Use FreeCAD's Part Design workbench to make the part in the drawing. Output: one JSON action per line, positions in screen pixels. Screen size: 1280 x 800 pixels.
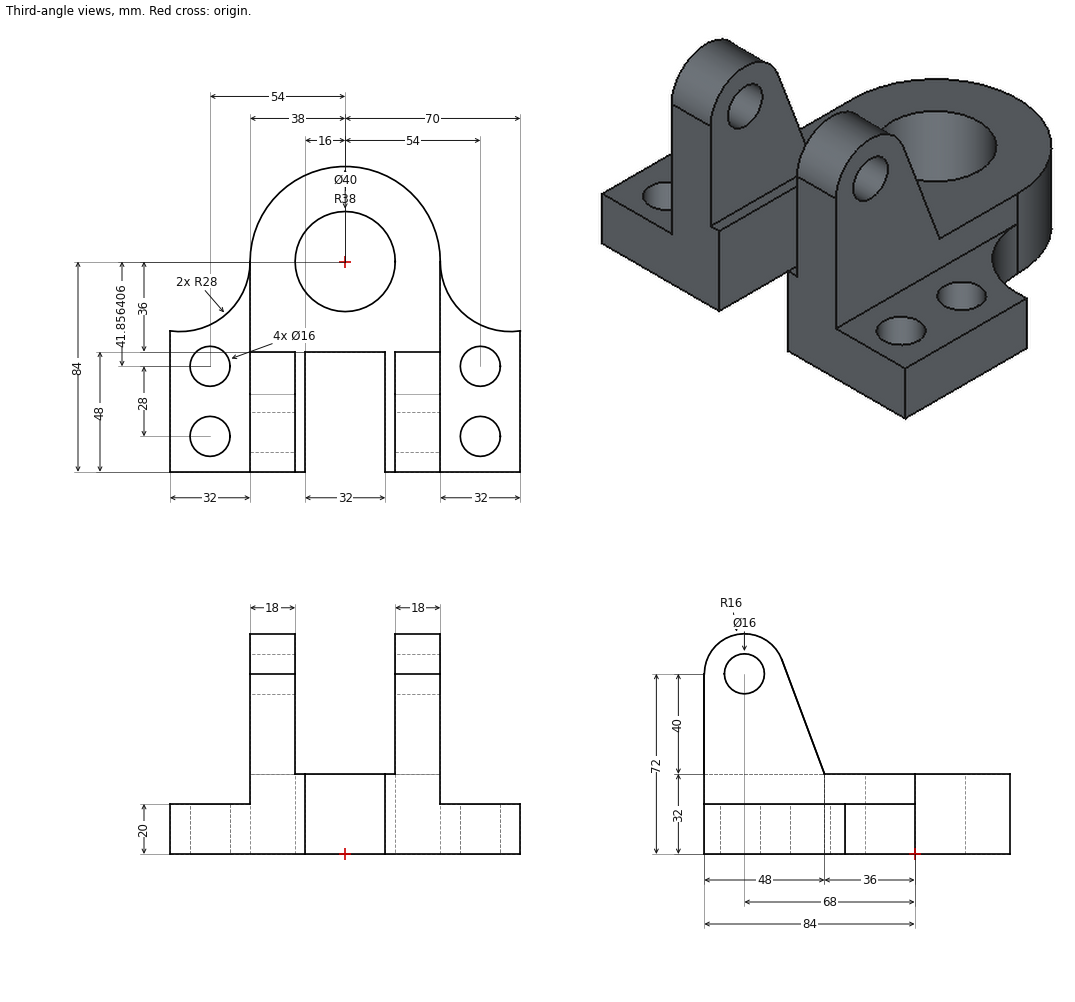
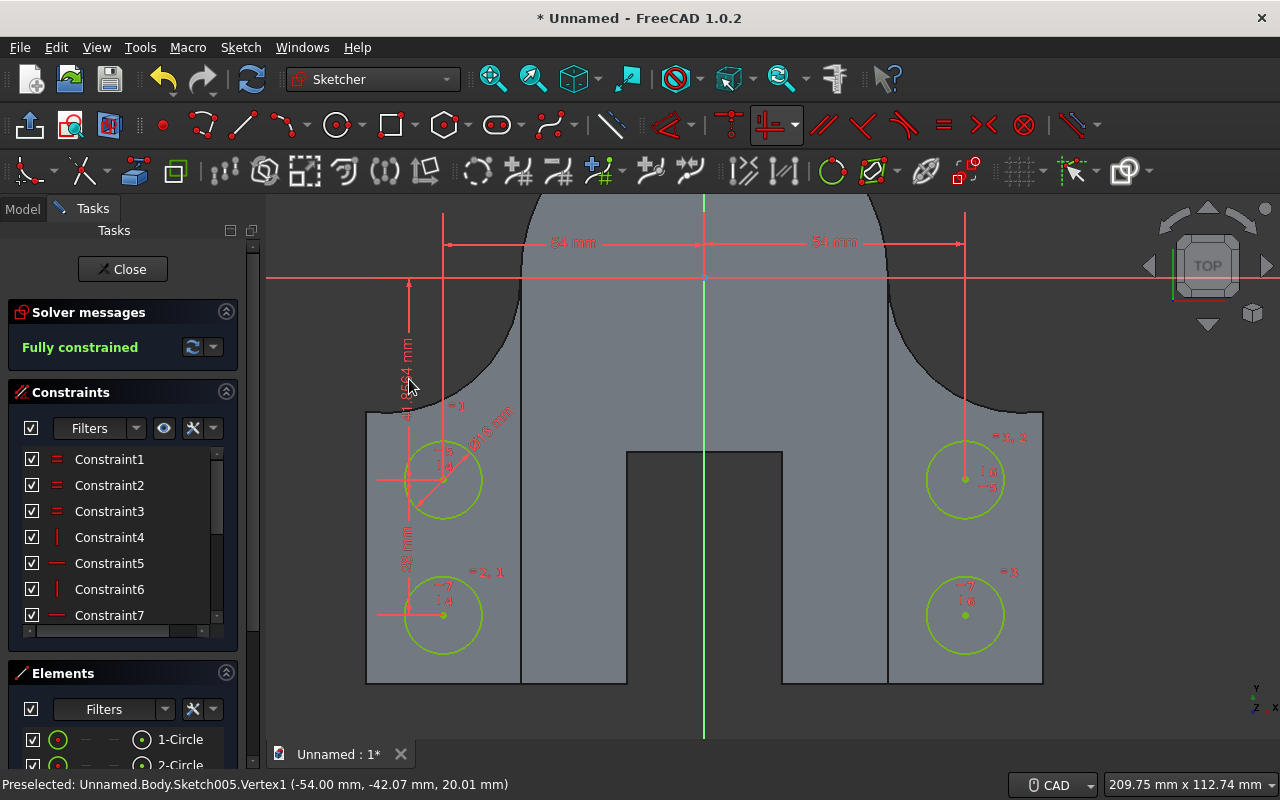
{"action": "left_click", "coordinate": [123, 269]}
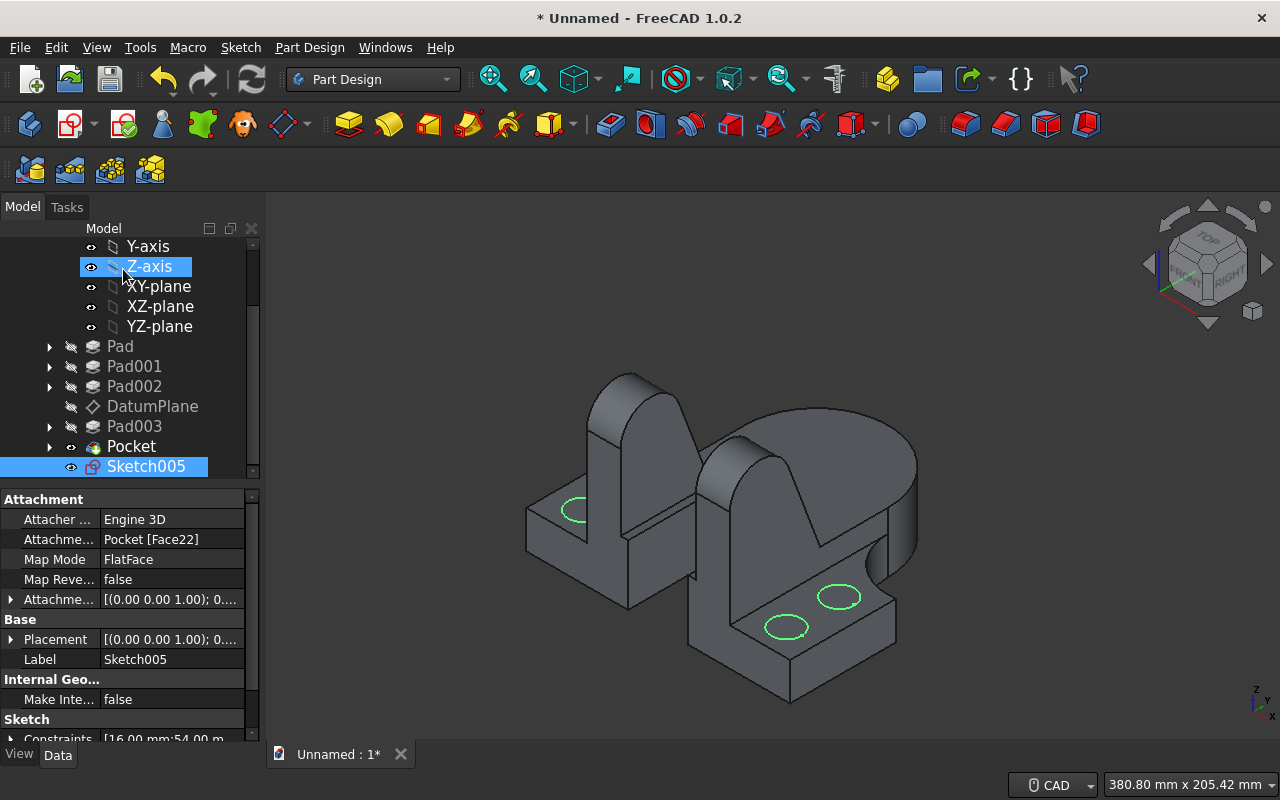
{"action": "left_click", "coordinate": [612, 124]}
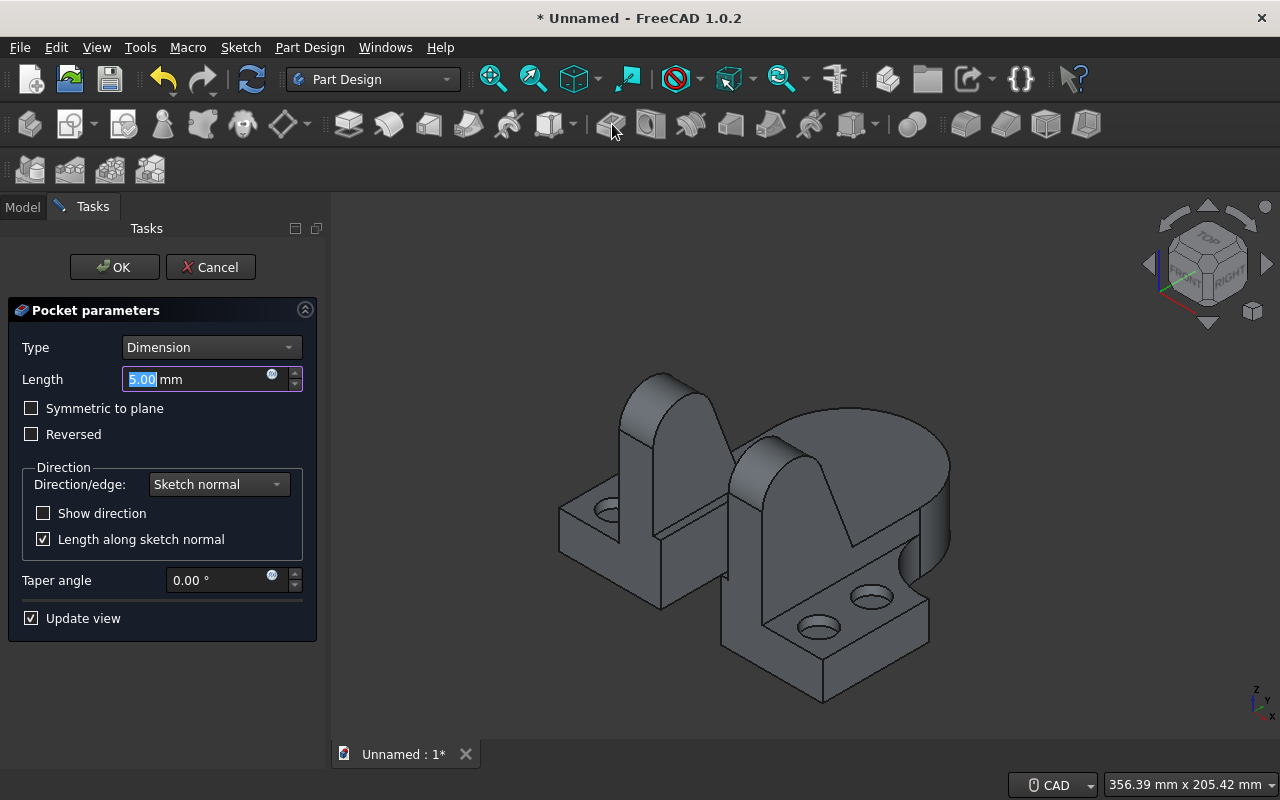
{"action": "left_click", "coordinate": [212, 348]}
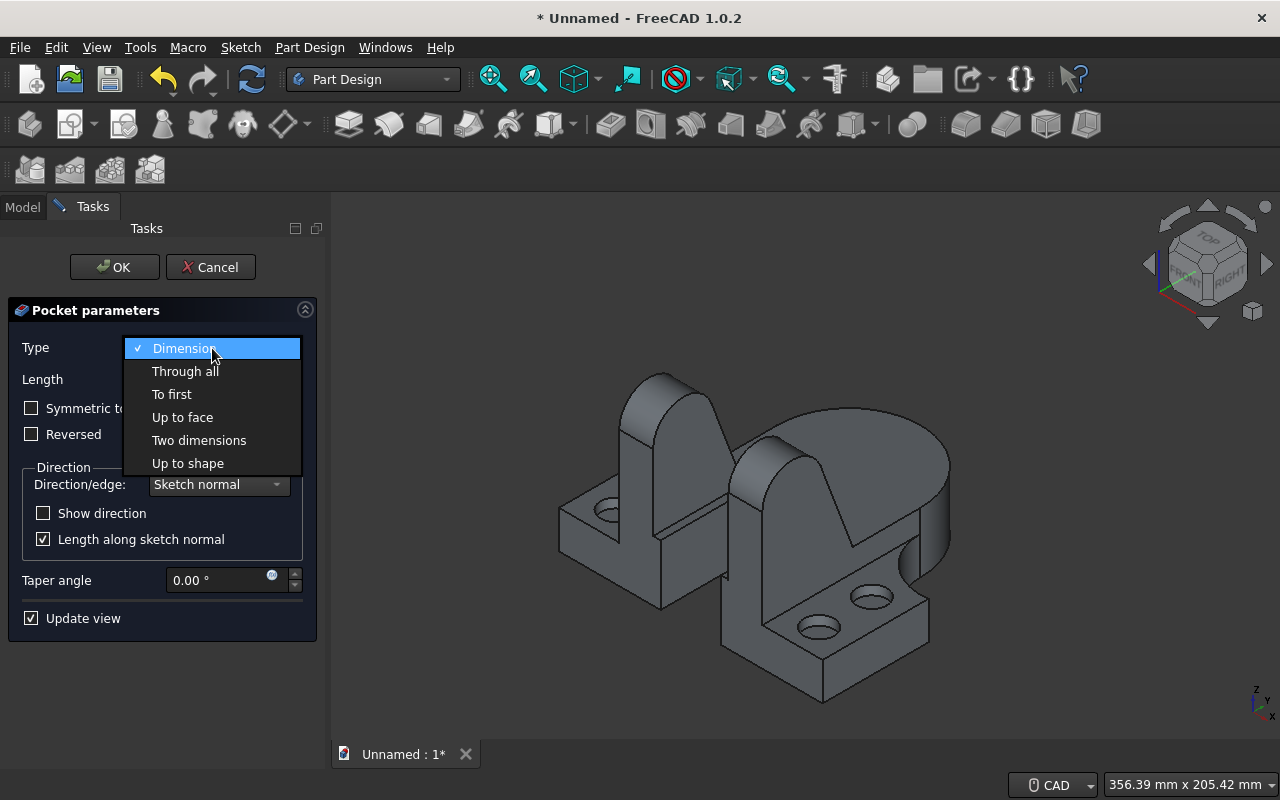
{"action": "left_click", "coordinate": [212, 372]}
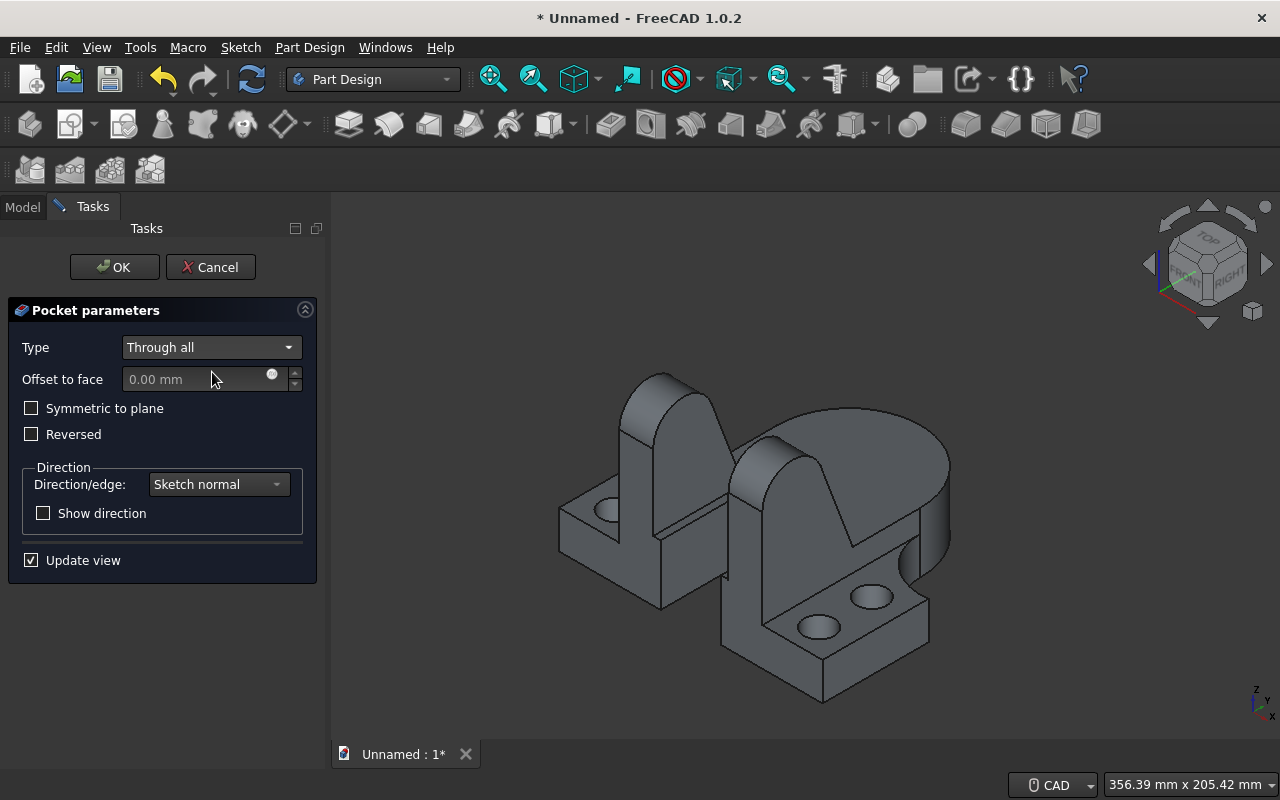
{"action": "left_click", "coordinate": [115, 267]}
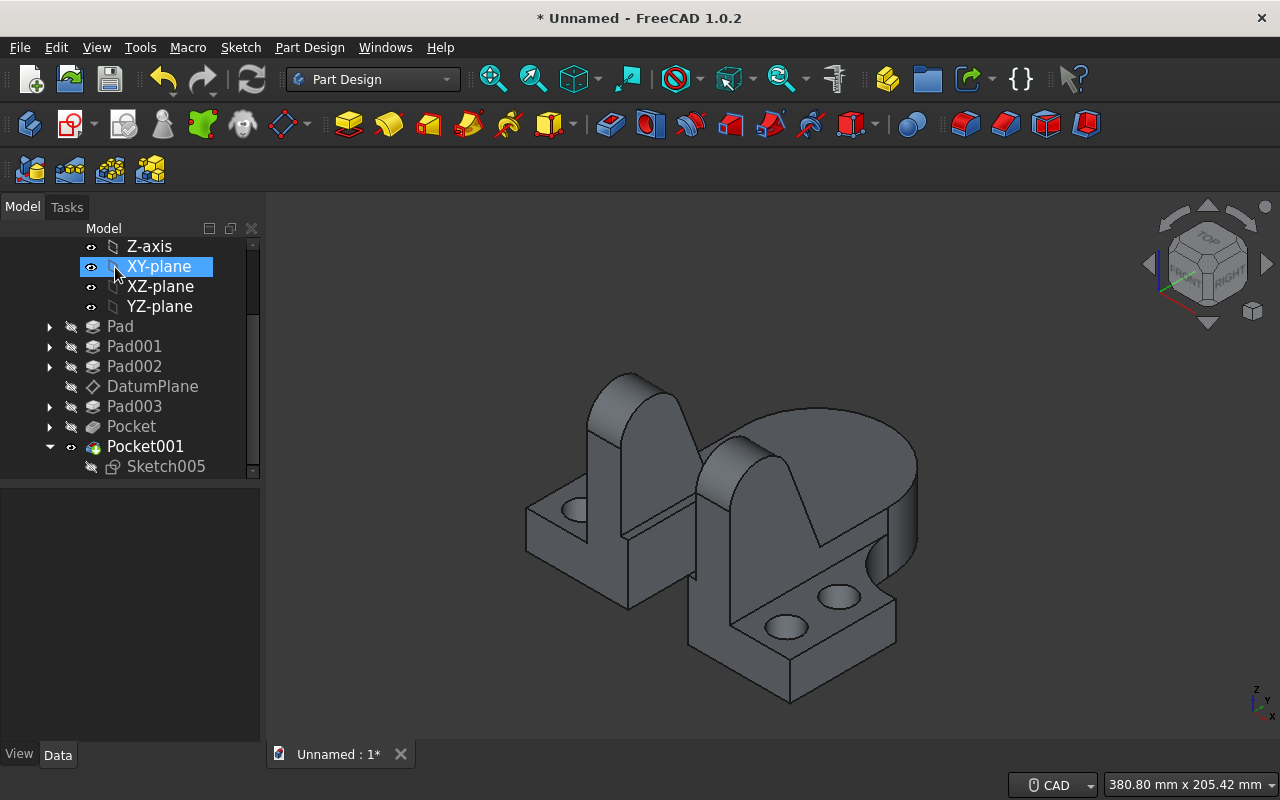
{"action": "key", "text": "6"}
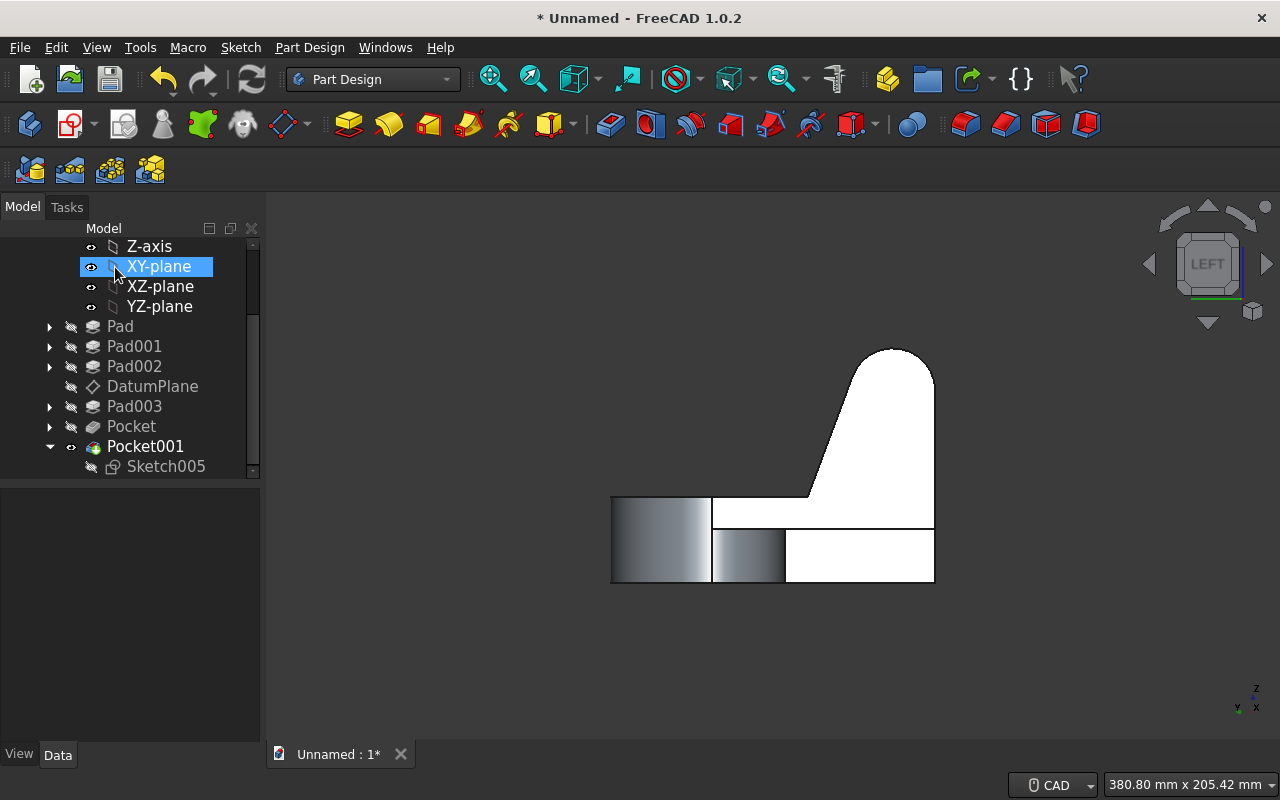
{"action": "left_click", "coordinate": [494, 80]}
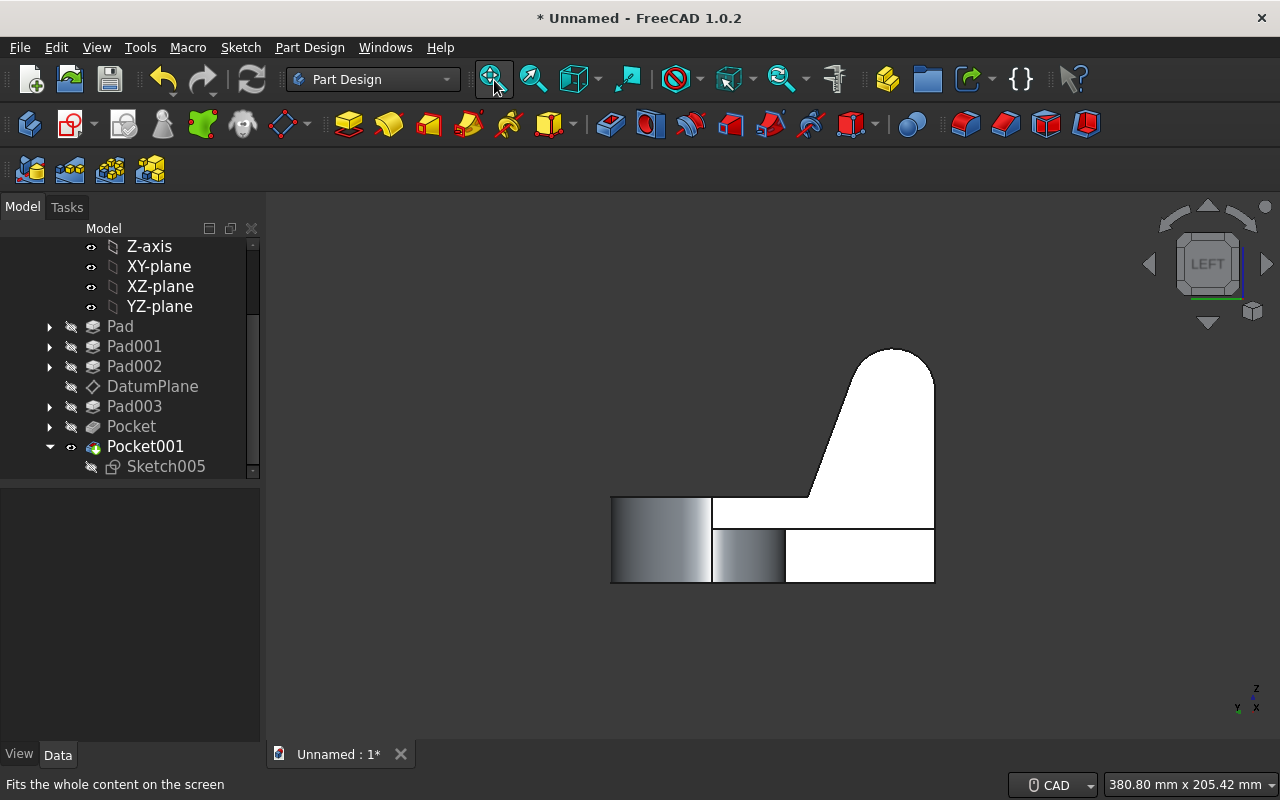
{"action": "left_click", "coordinate": [887, 438]}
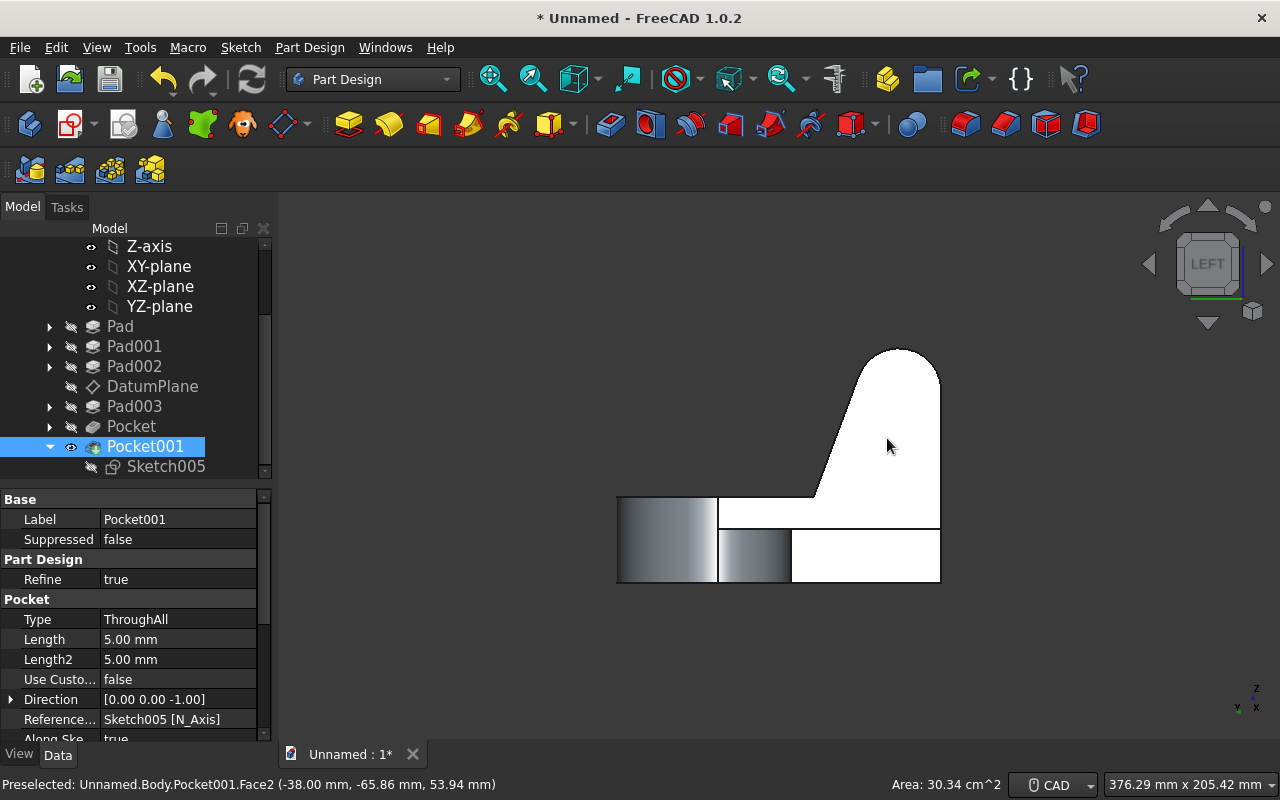
{"action": "left_click", "coordinate": [70, 124]}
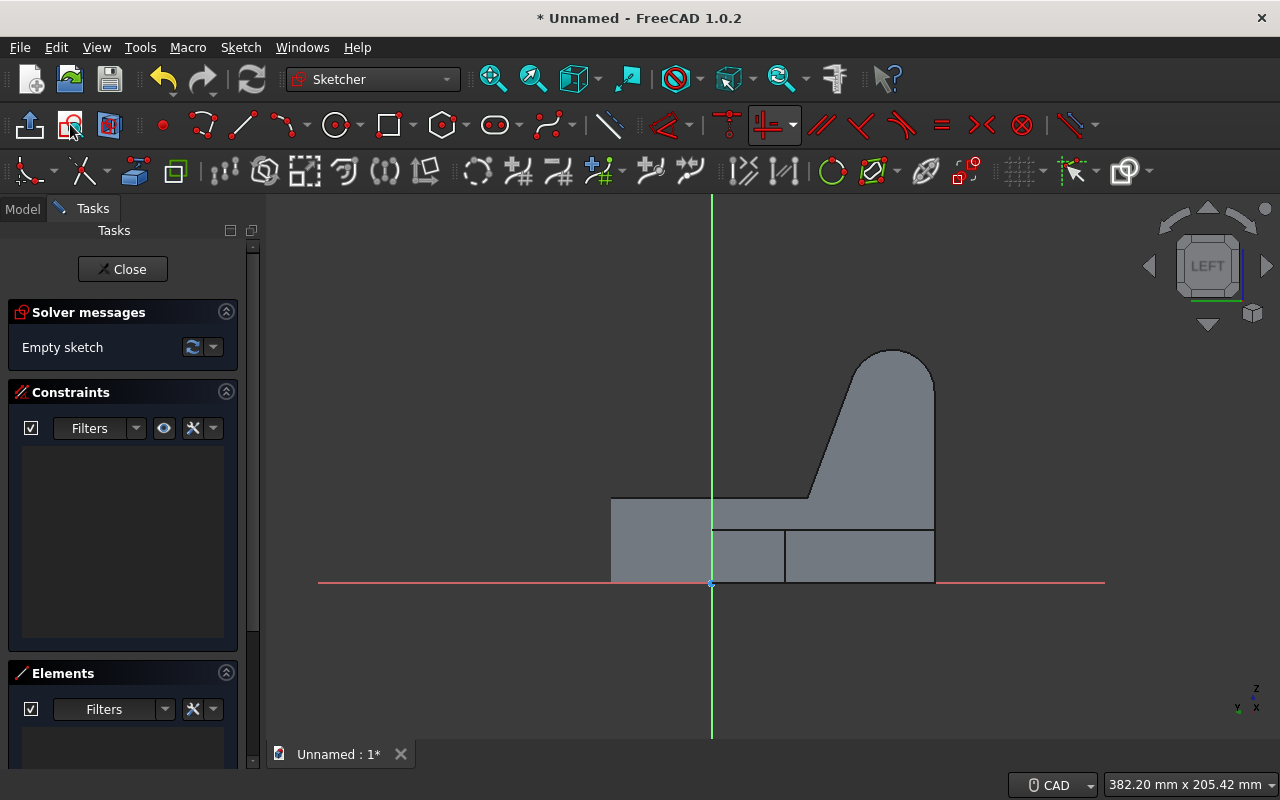
{"action": "scroll", "coordinate": [922, 381], "scroll_direction": "up", "scroll_amount": 10}